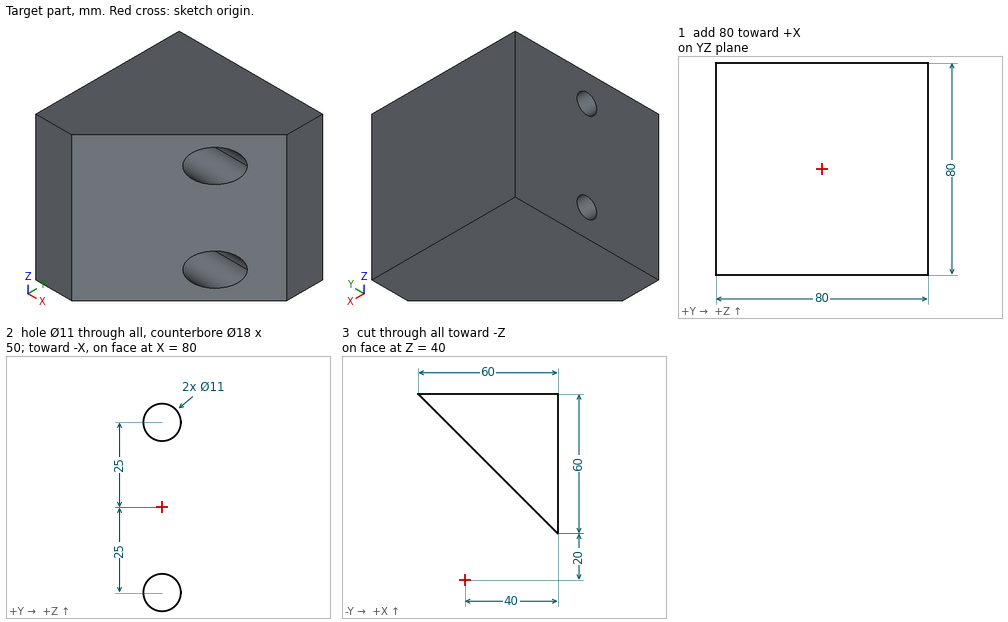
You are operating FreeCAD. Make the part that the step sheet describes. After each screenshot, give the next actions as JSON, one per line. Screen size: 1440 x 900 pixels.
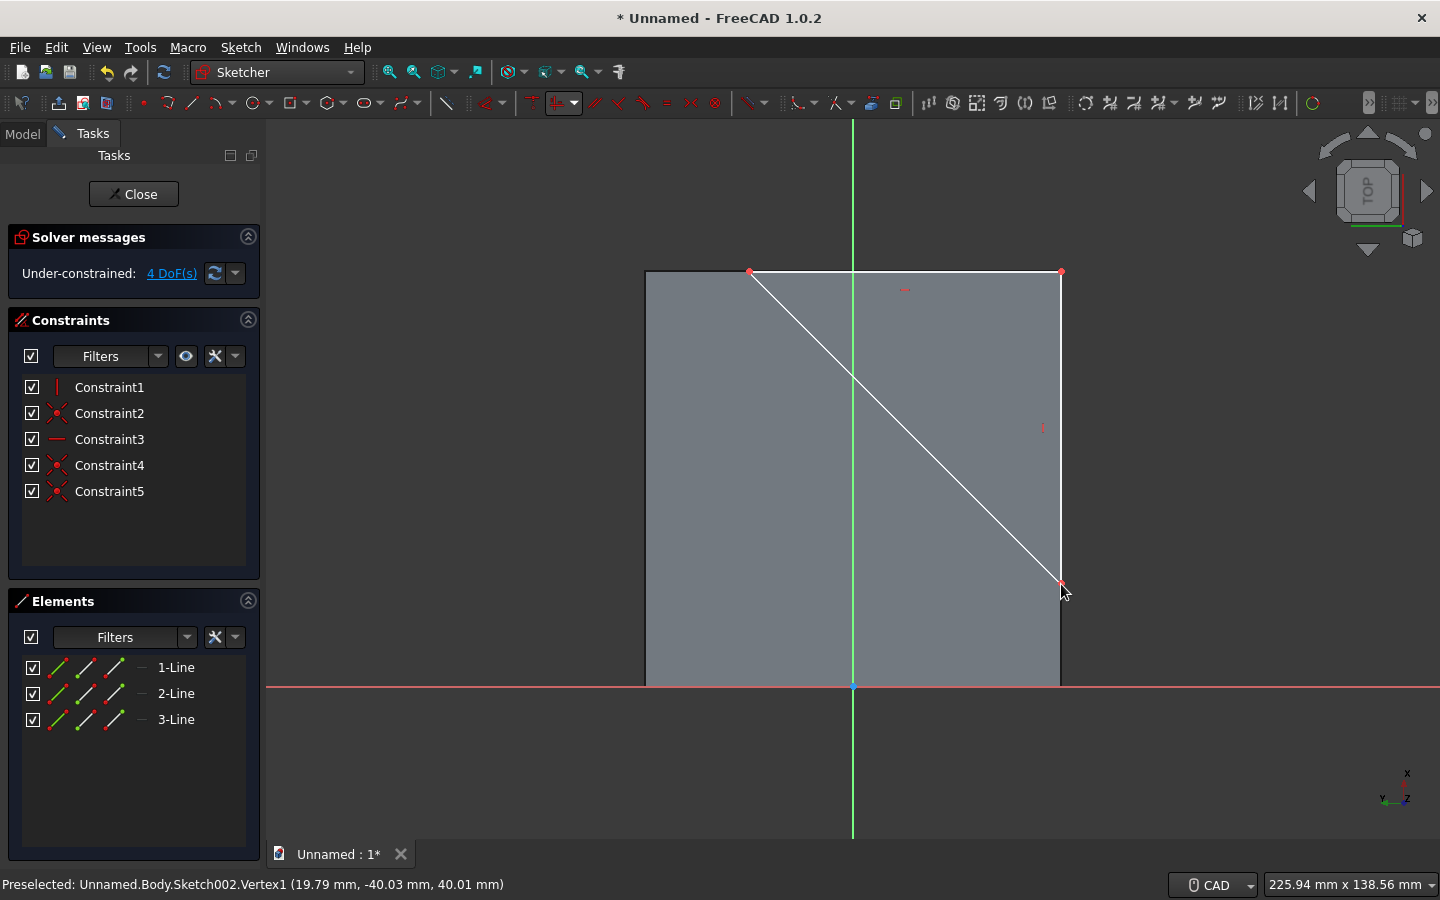
{"action": "left_click", "coordinate": [486, 104]}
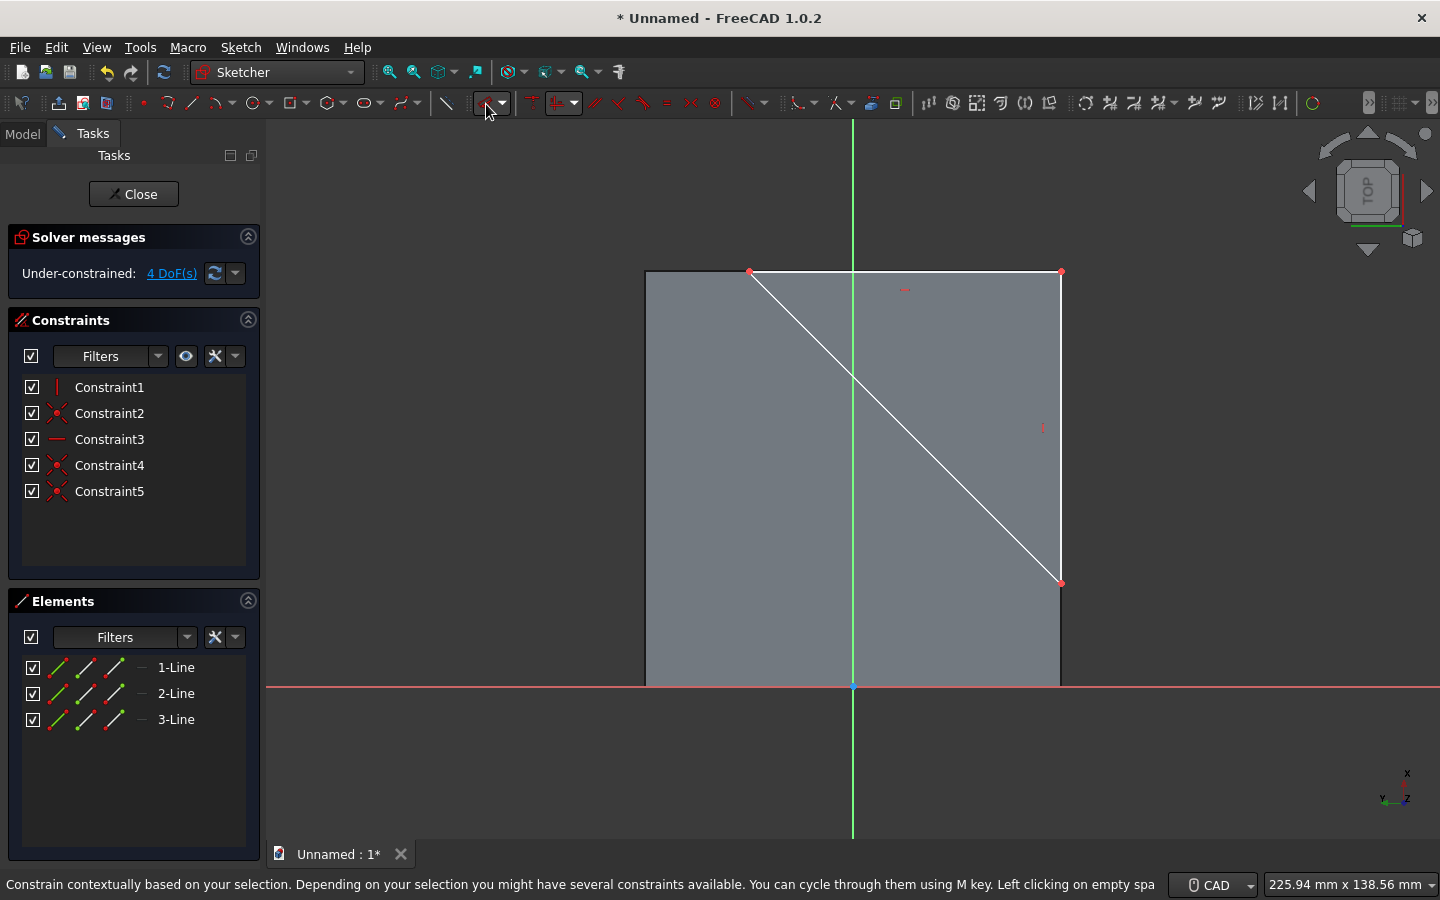
{"action": "left_click", "coordinate": [1061, 490]}
{"action": "left_click", "coordinate": [1095, 428]}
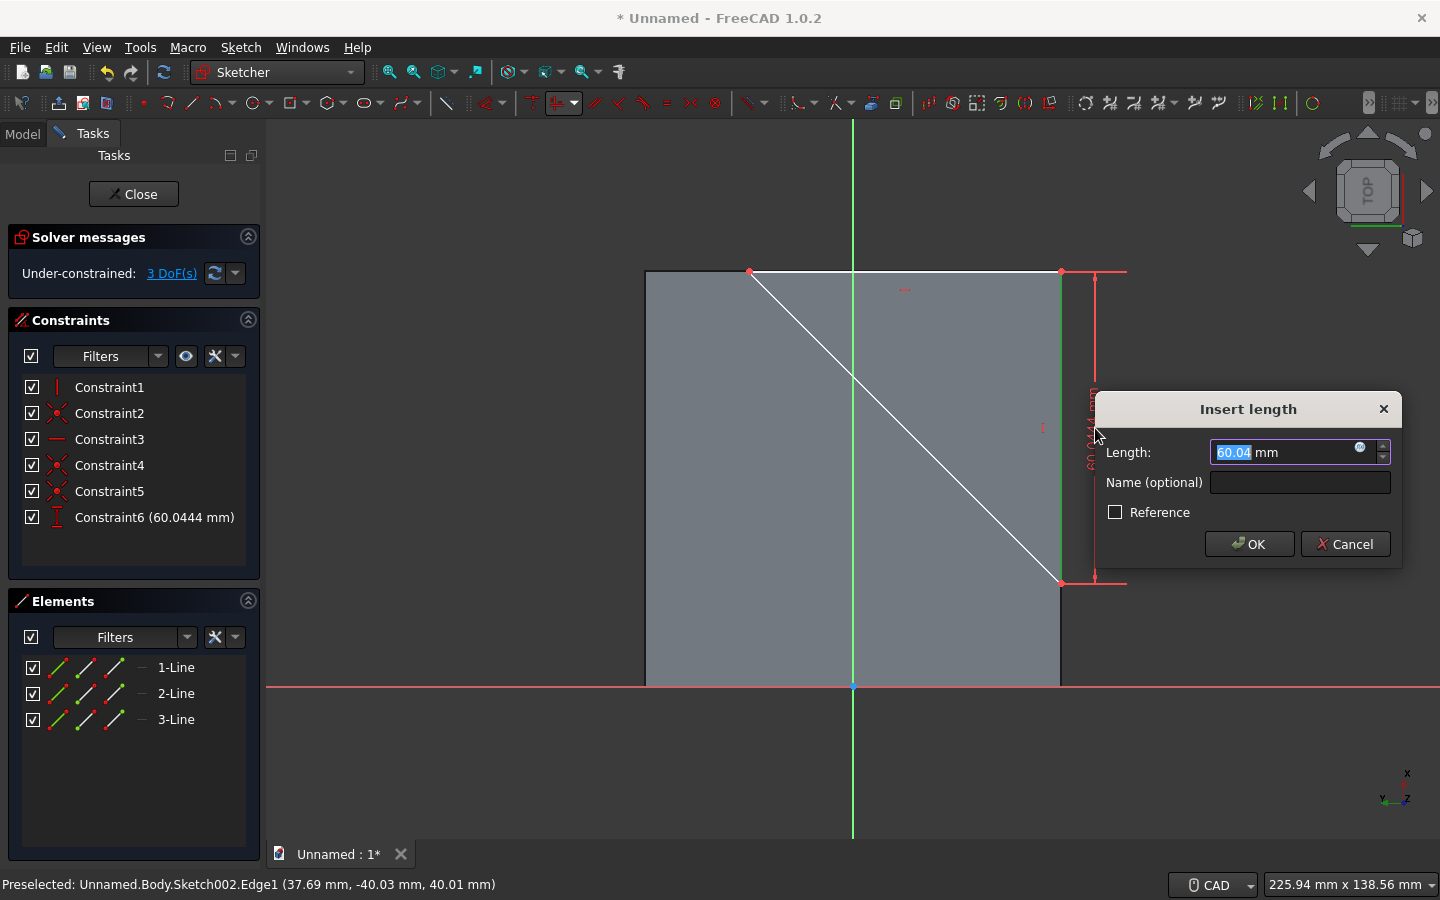
{"action": "type", "text": "60"}
{"action": "key", "text": "Return"}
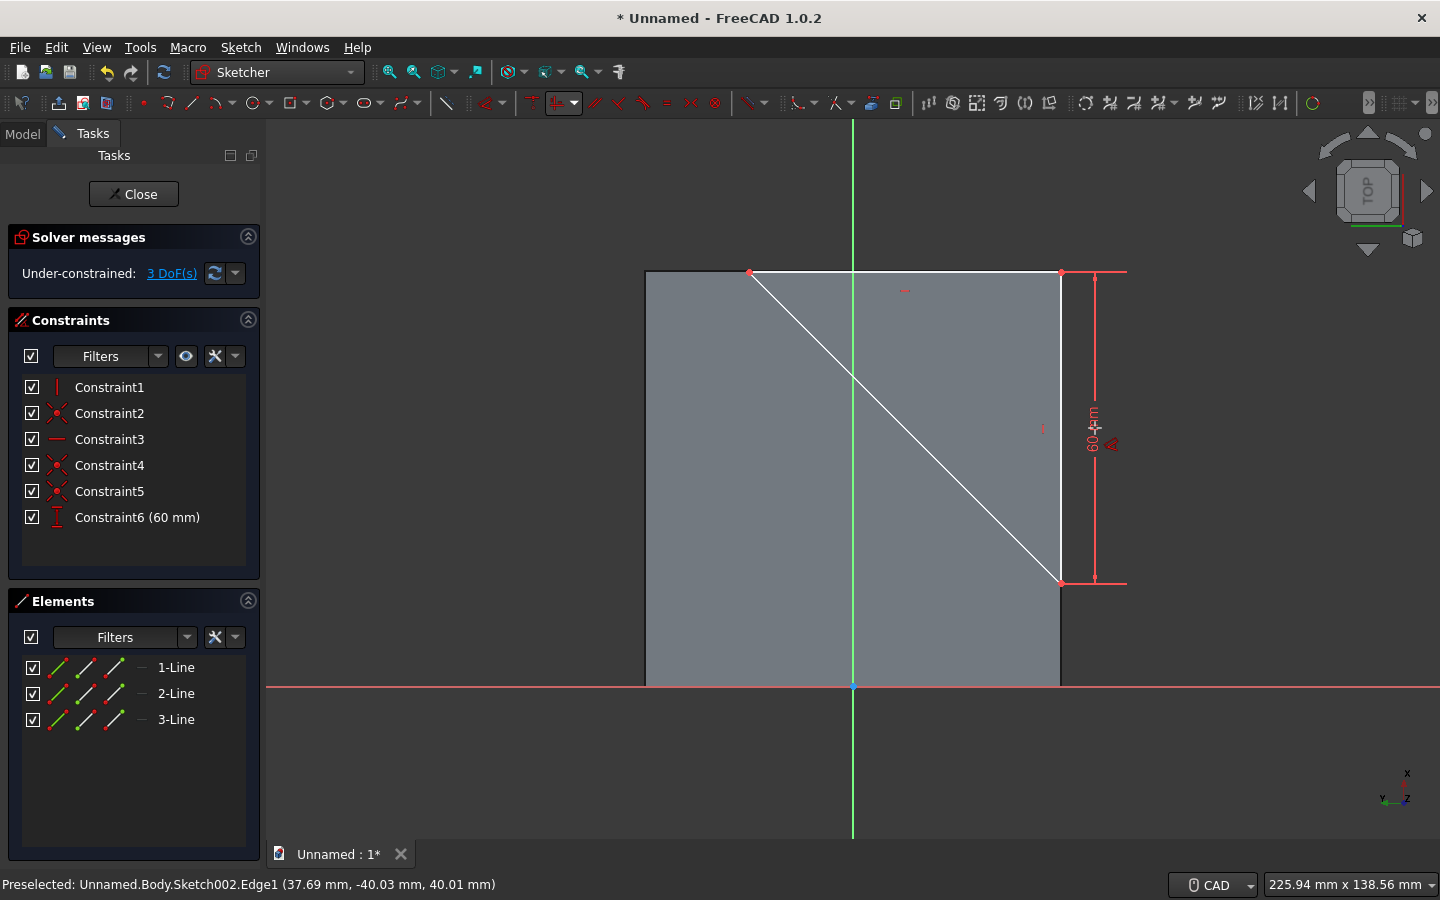
{"action": "left_click", "coordinate": [967, 272]}
{"action": "left_click", "coordinate": [905, 238]}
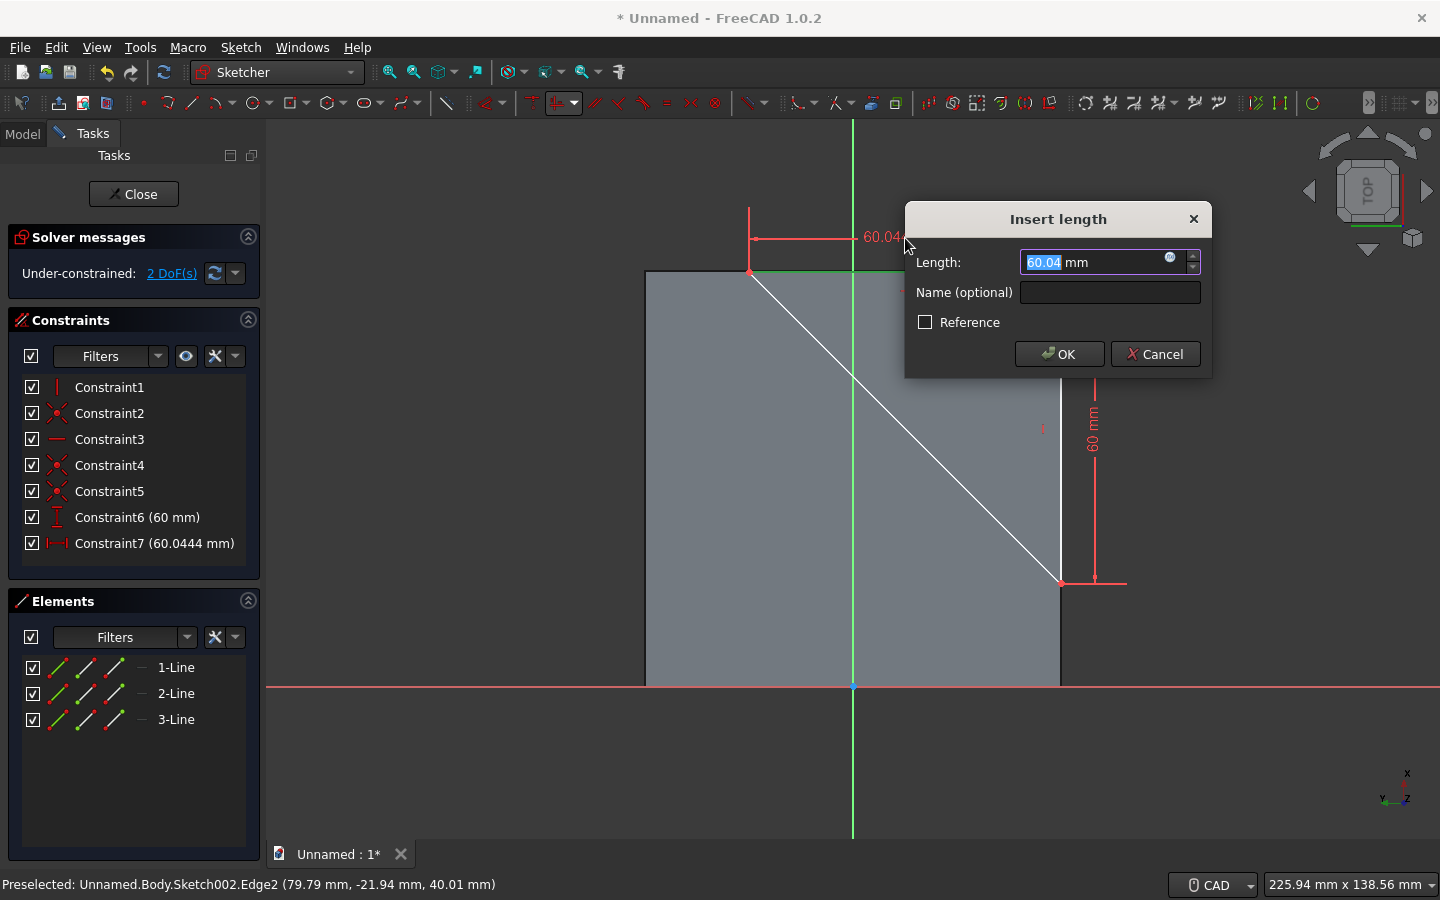
{"action": "type", "text": "60"}
{"action": "key", "text": "Return"}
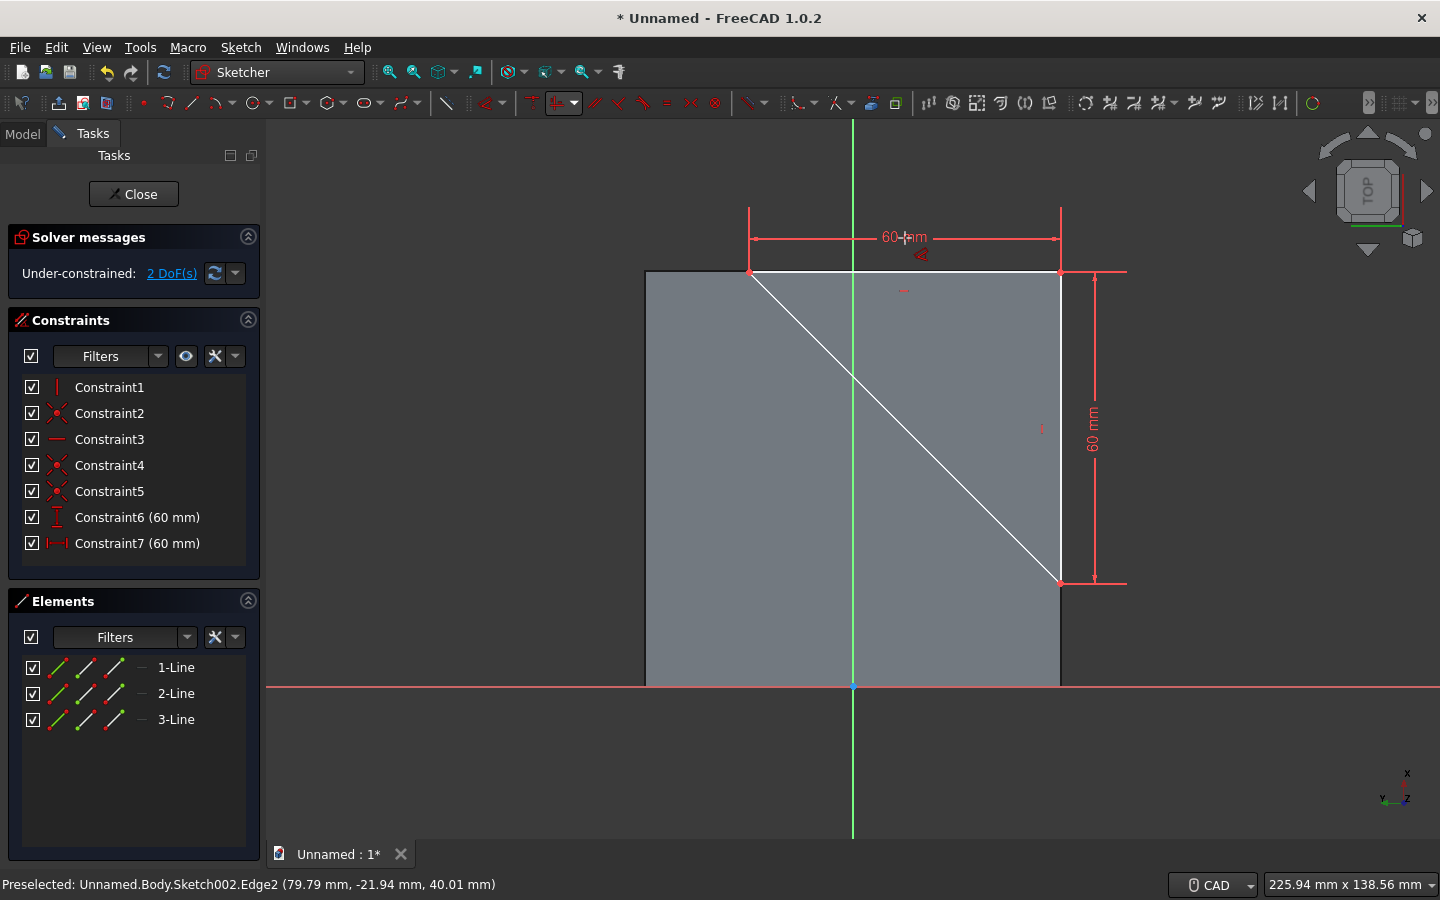
{"action": "left_click", "coordinate": [1061, 584]}
{"action": "left_click", "coordinate": [957, 721]}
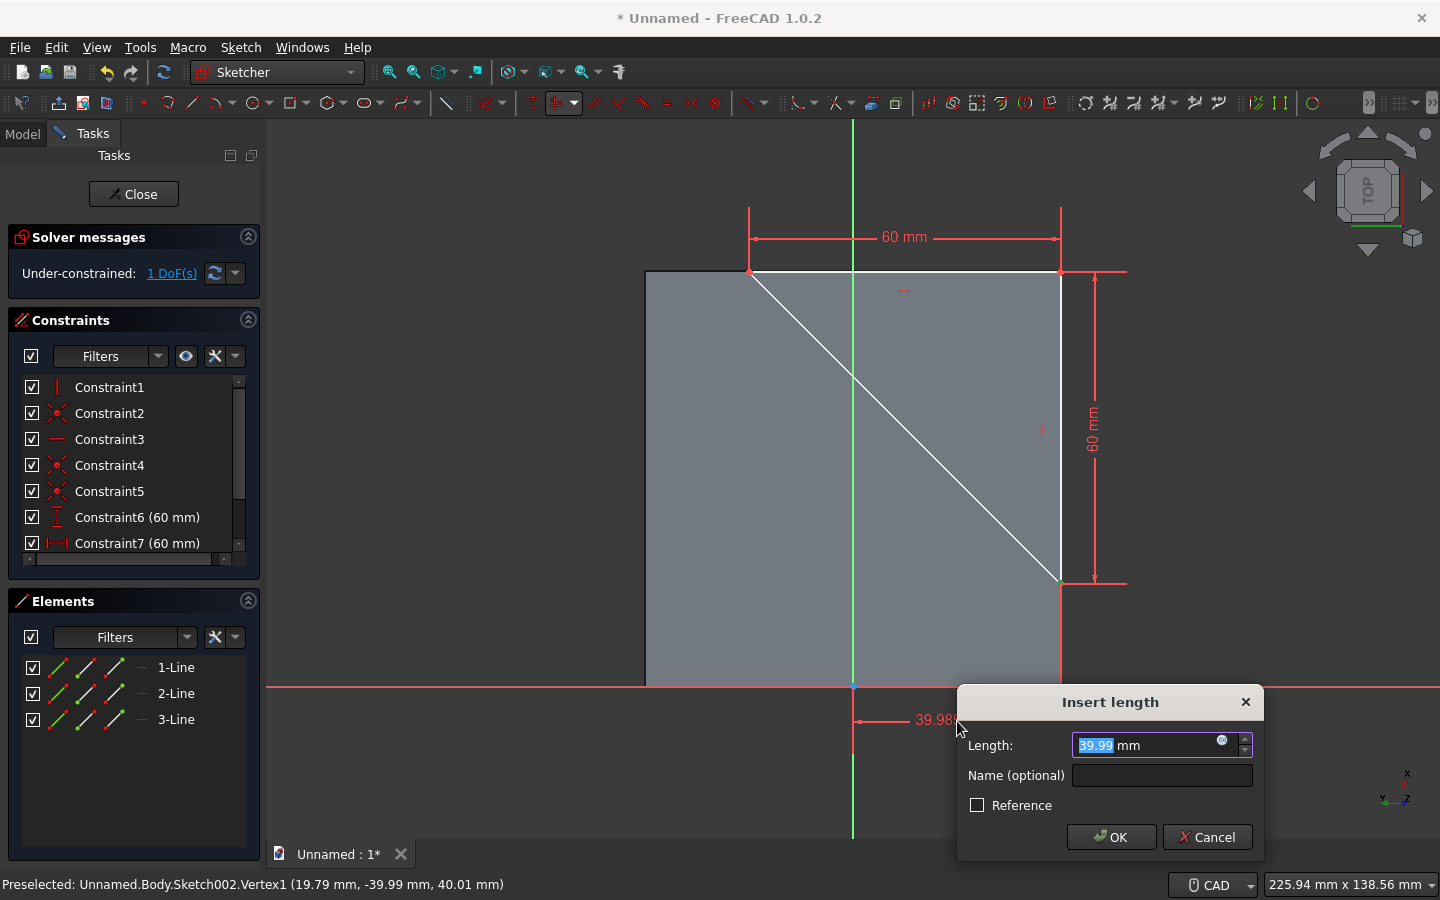
{"action": "type", "text": "40"}
{"action": "key", "text": "Return"}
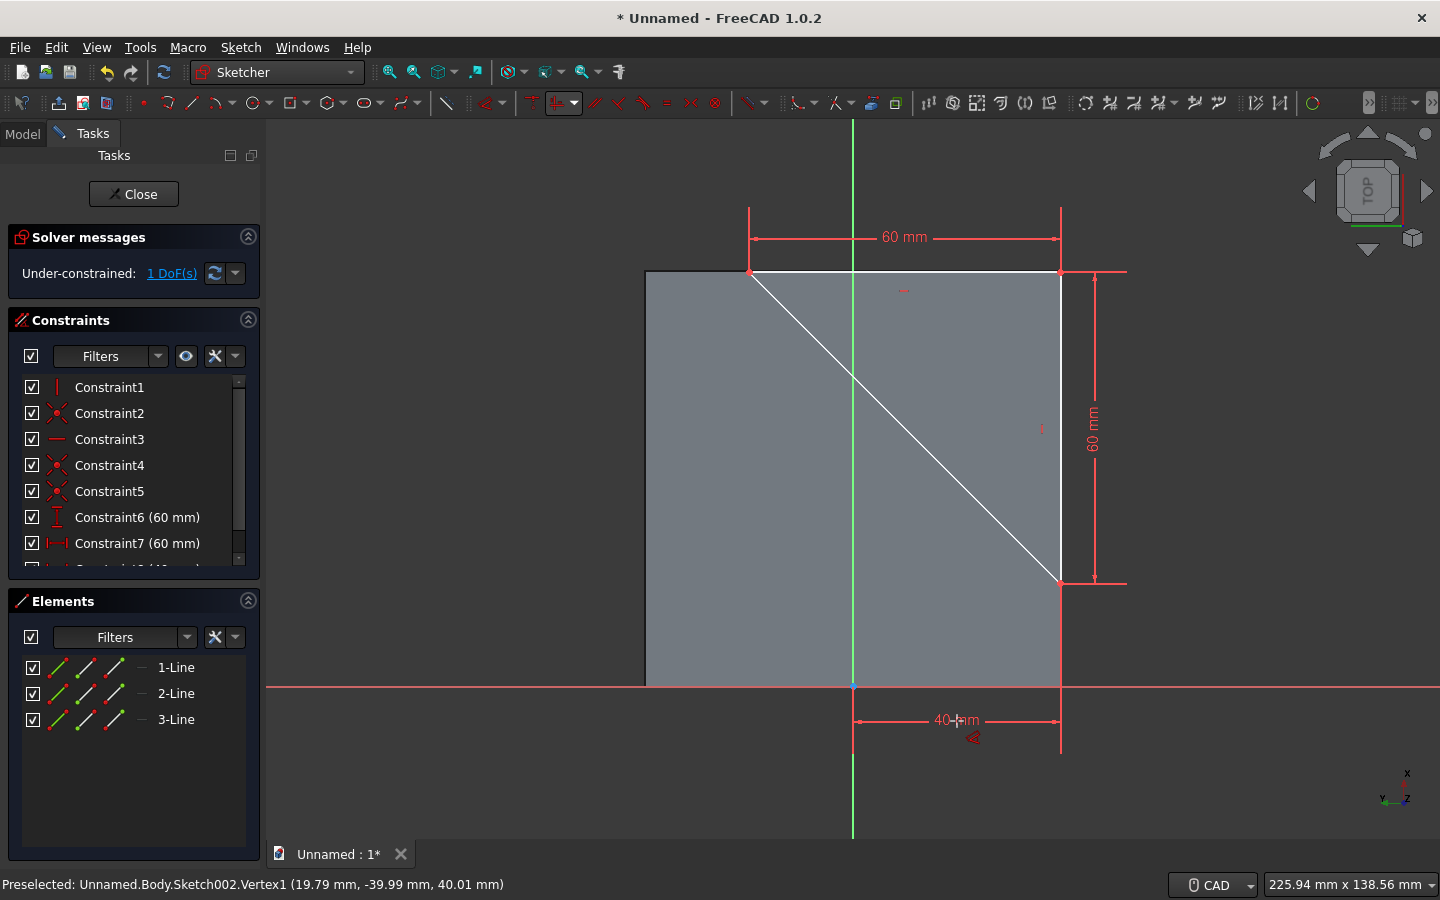
{"action": "left_click", "coordinate": [1061, 584]}
{"action": "left_click", "coordinate": [1095, 635]}